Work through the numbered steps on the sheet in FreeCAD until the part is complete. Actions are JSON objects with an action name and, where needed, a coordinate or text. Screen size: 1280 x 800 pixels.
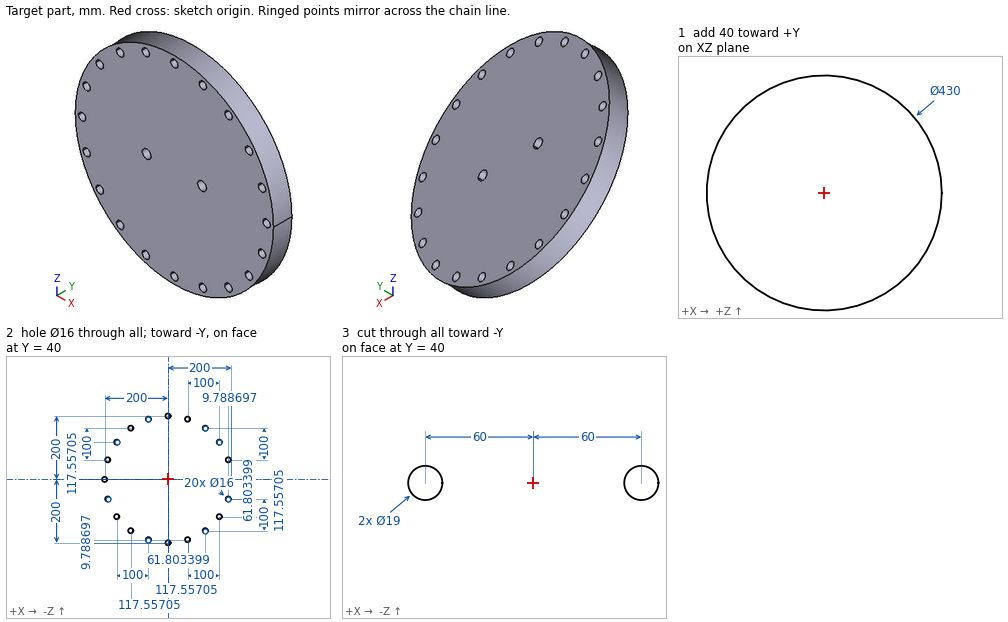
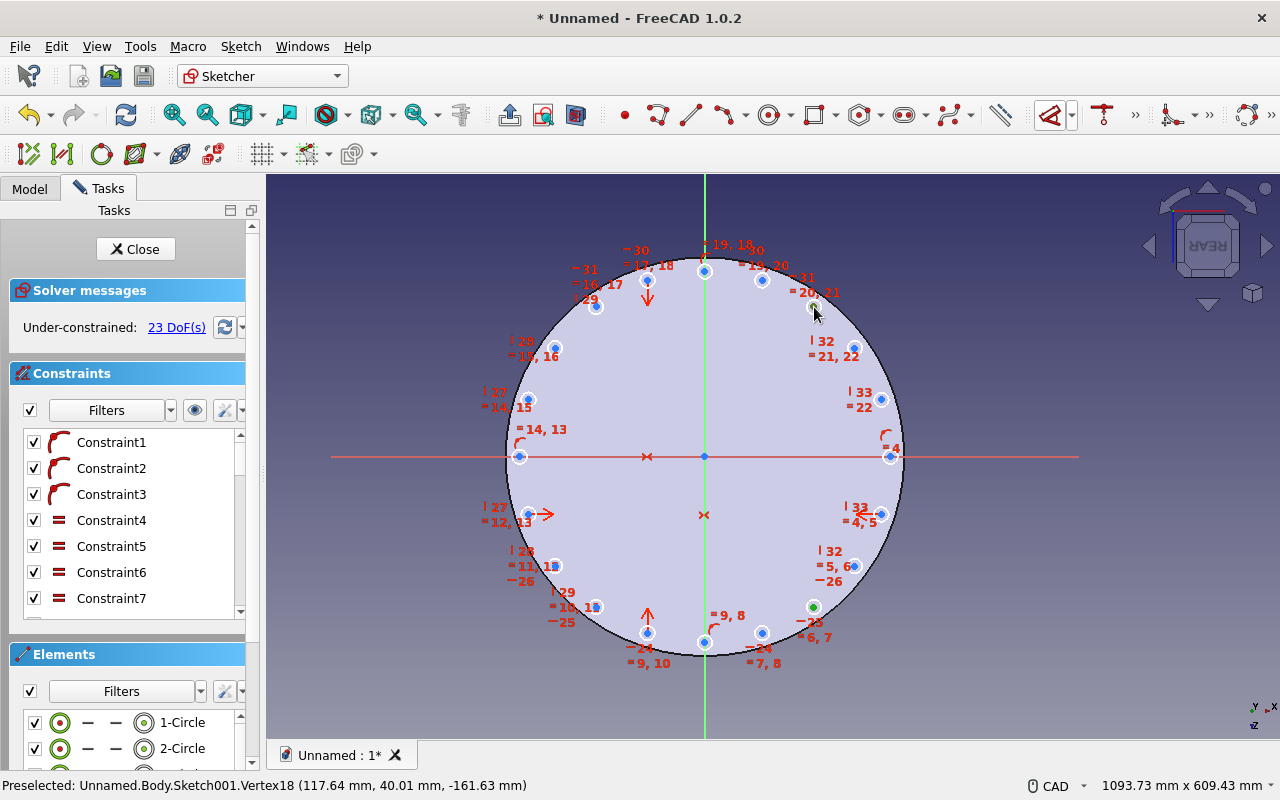
{"action": "left_click", "coordinate": [353, 457]}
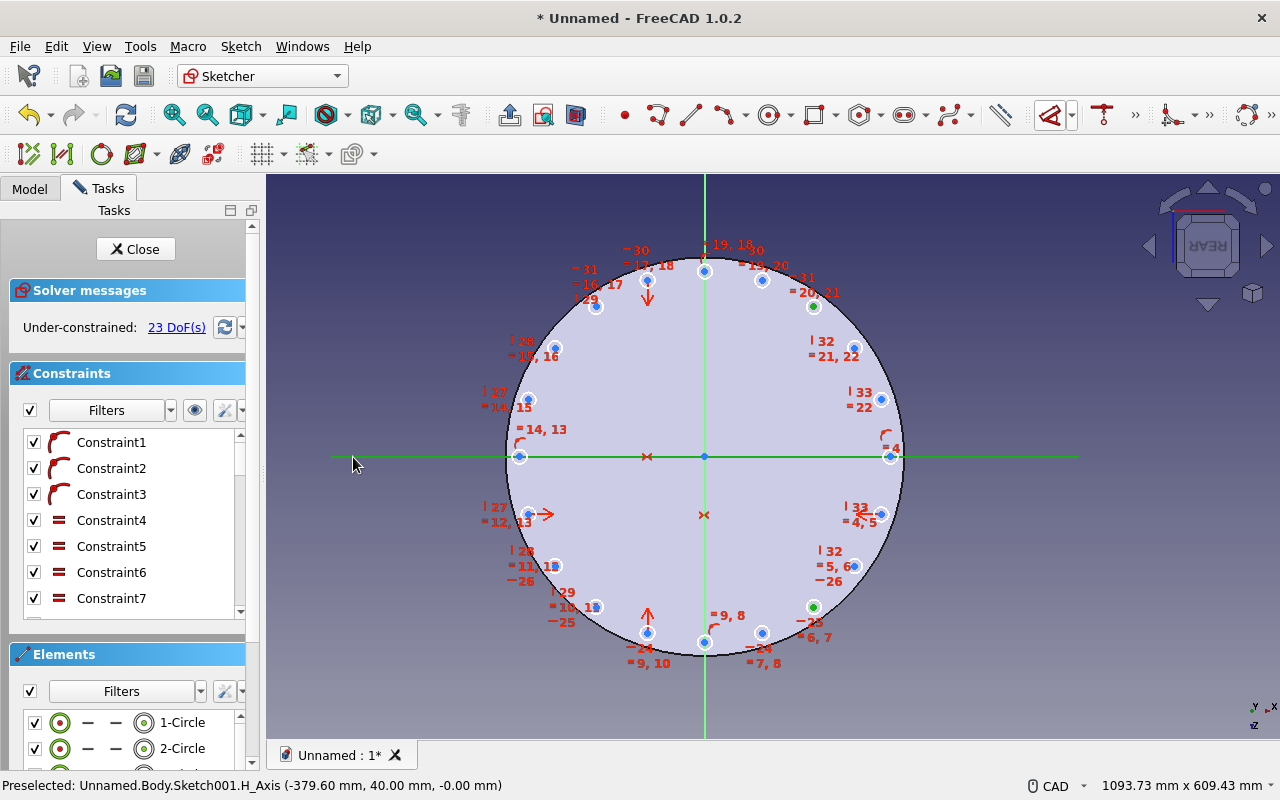
{"action": "key", "text": "s"}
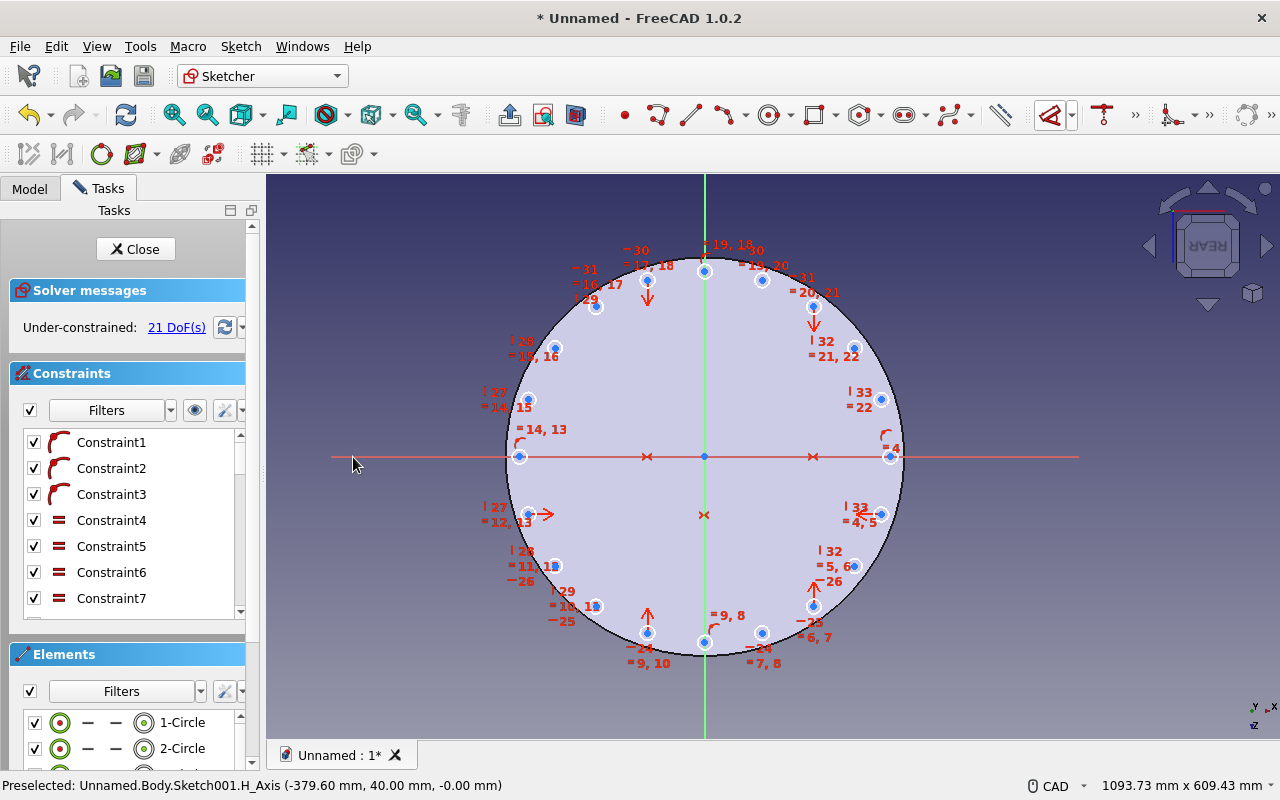
{"action": "scroll", "coordinate": [555, 348], "scroll_direction": "up", "scroll_amount": 4}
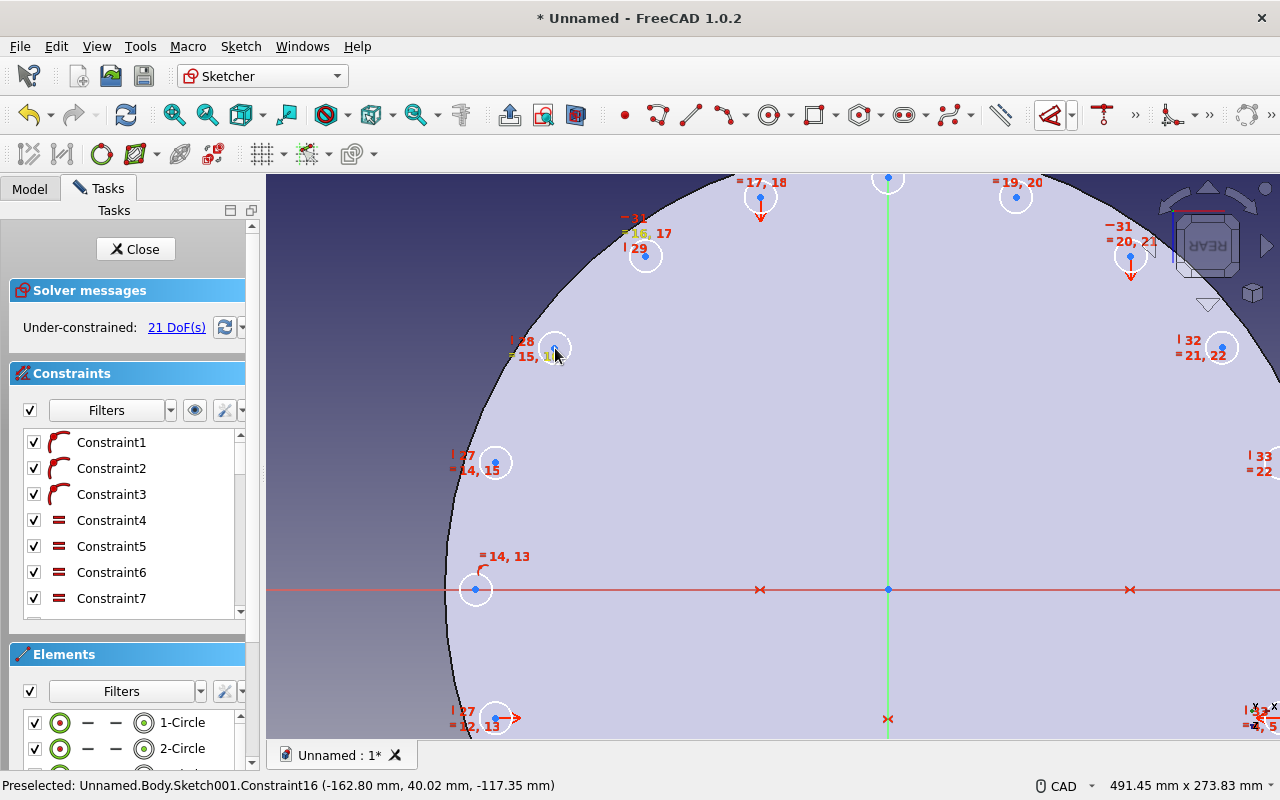
{"action": "scroll", "coordinate": [555, 348], "scroll_direction": "up", "scroll_amount": 4}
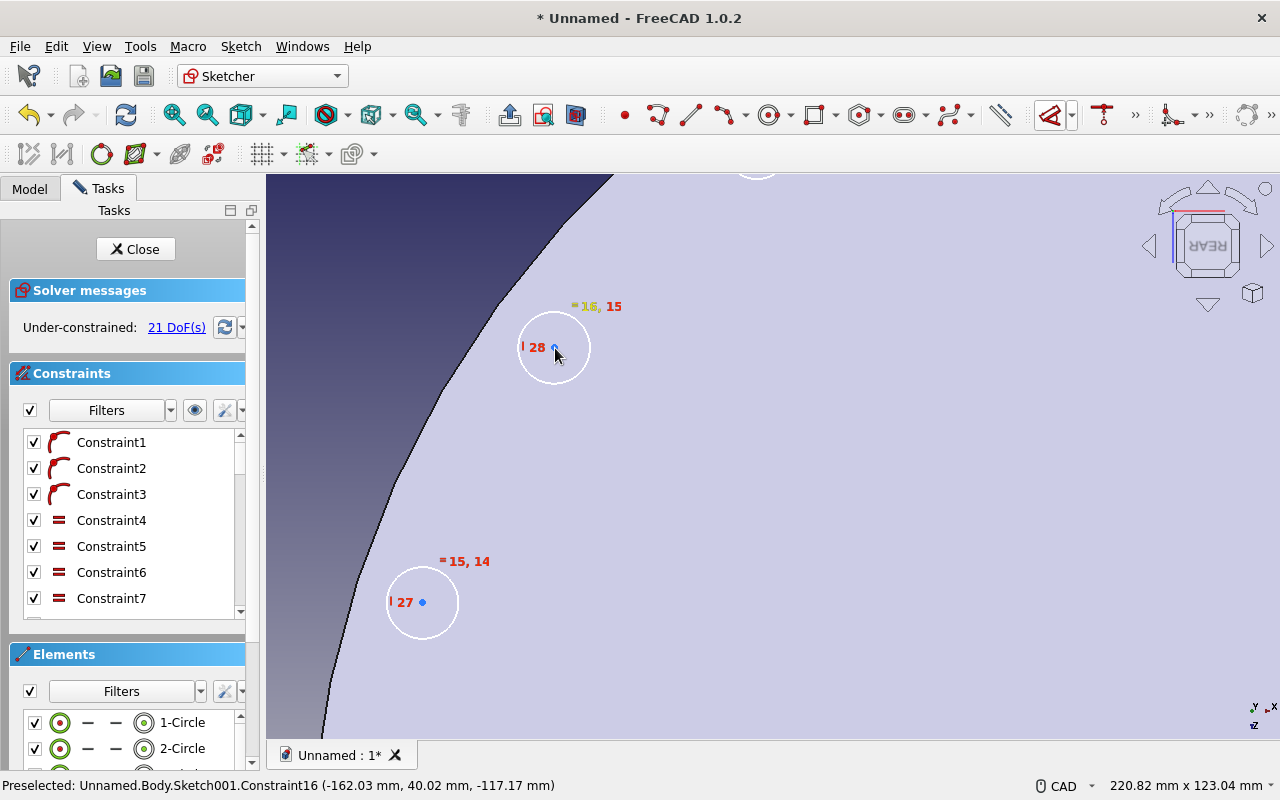
{"action": "left_click", "coordinate": [554, 348]}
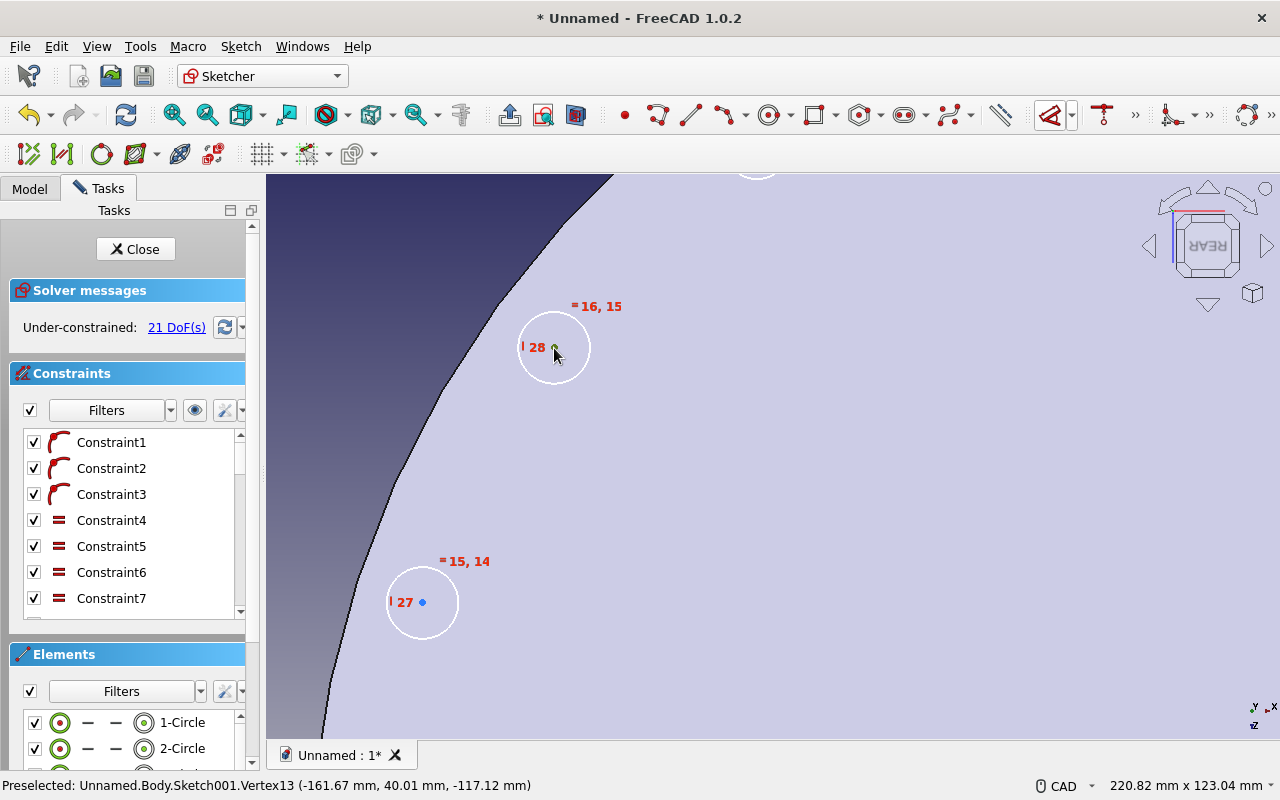
{"action": "scroll", "coordinate": [555, 348], "scroll_direction": "down", "scroll_amount": 8}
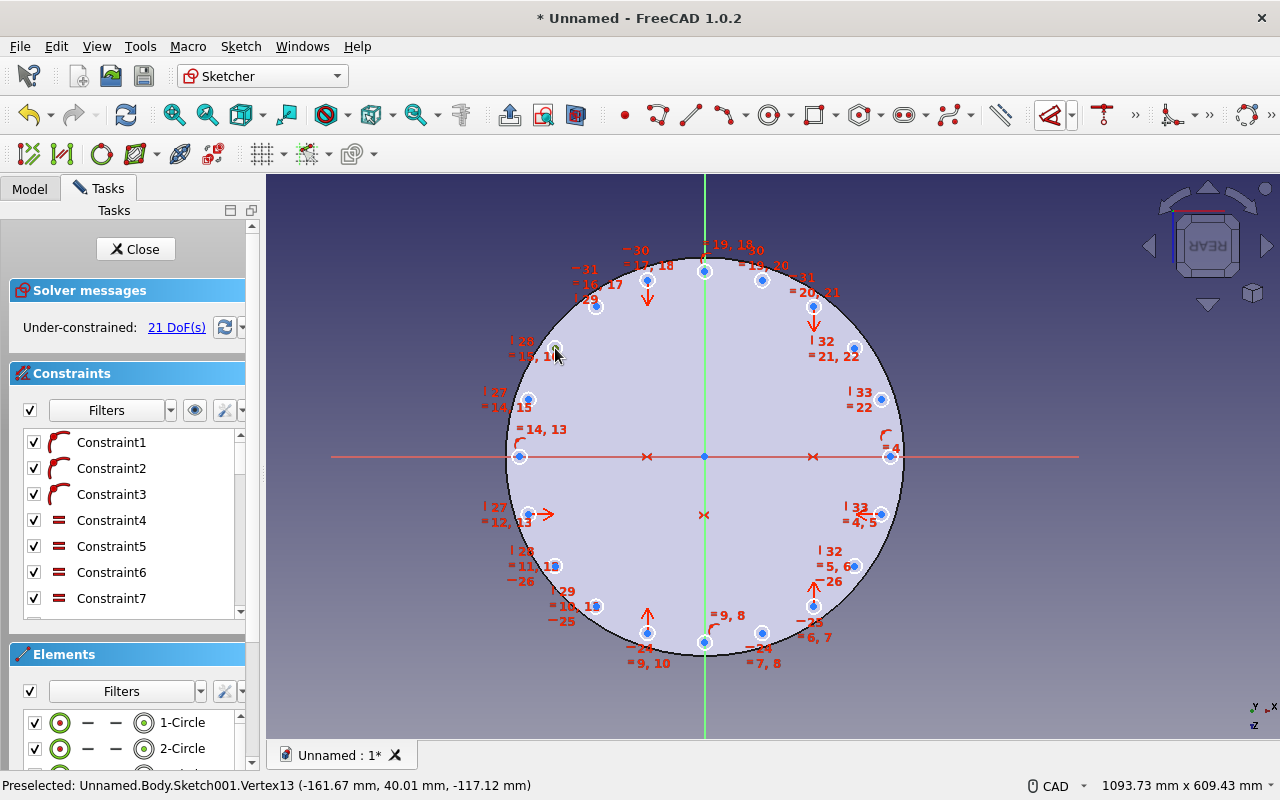
{"action": "scroll", "coordinate": [855, 348], "scroll_direction": "up", "scroll_amount": 4}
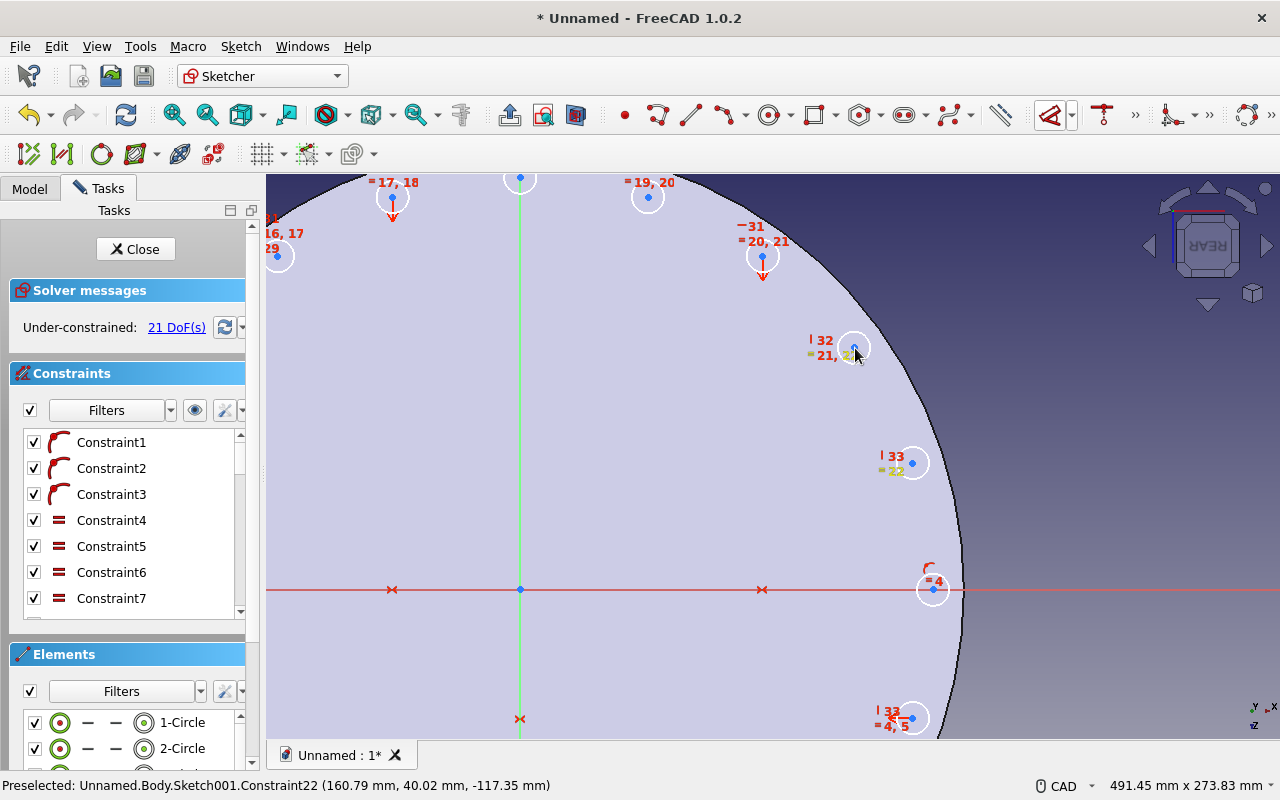
{"action": "scroll", "coordinate": [854, 348], "scroll_direction": "up", "scroll_amount": 4}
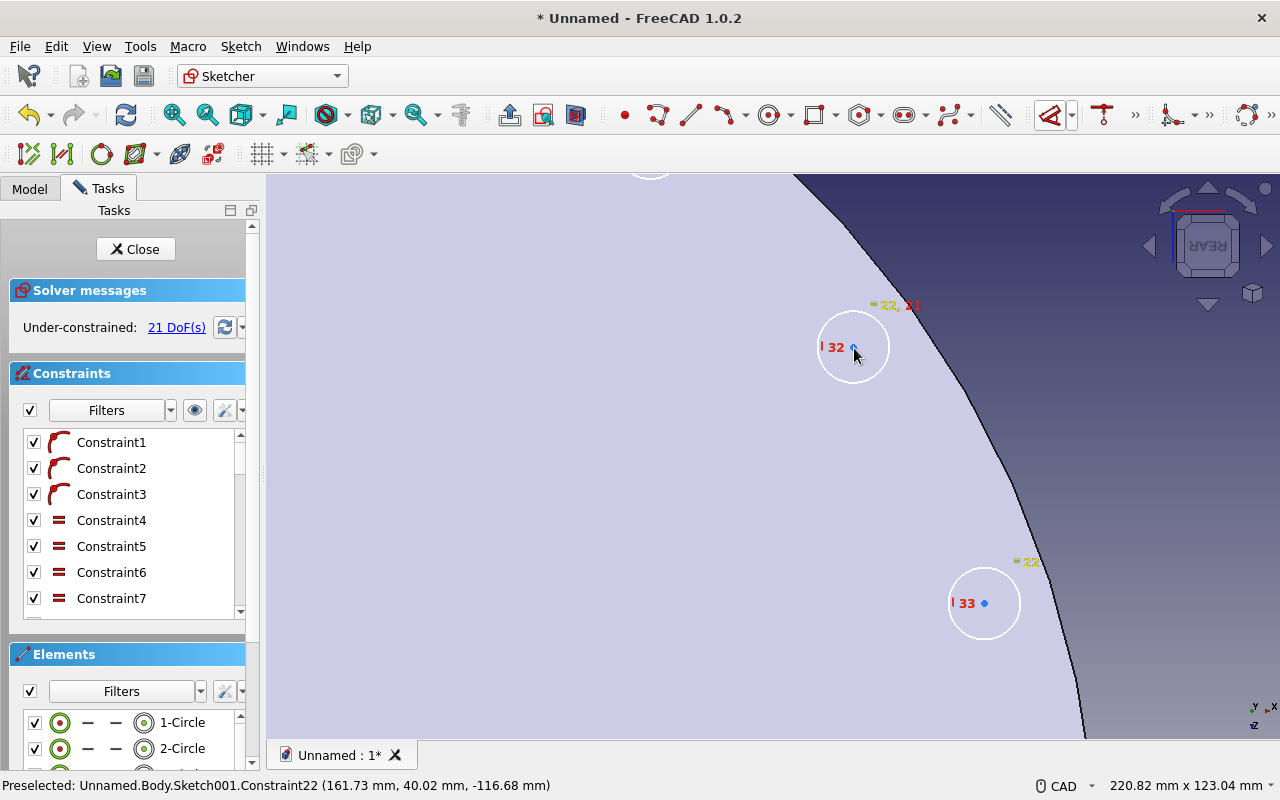
{"action": "left_click", "coordinate": [853, 347]}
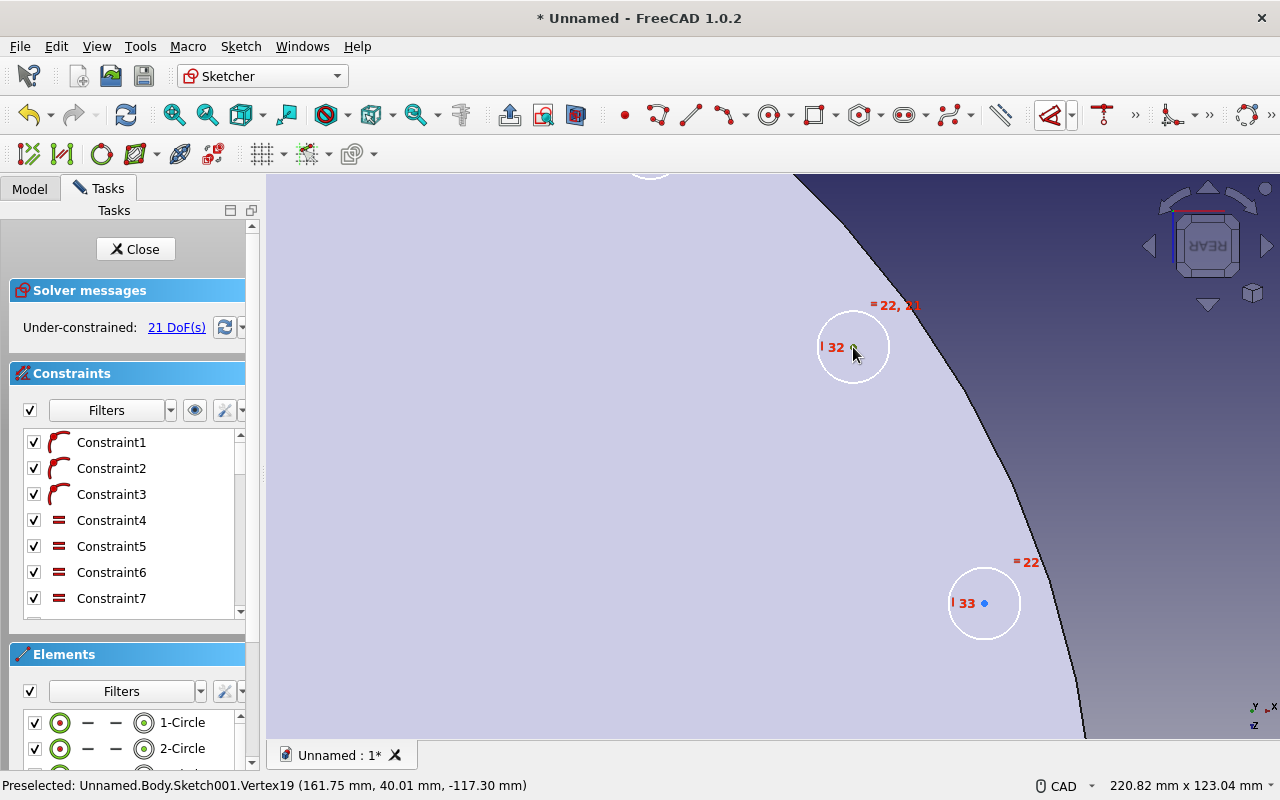
{"action": "scroll", "coordinate": [855, 348], "scroll_direction": "down", "scroll_amount": 8}